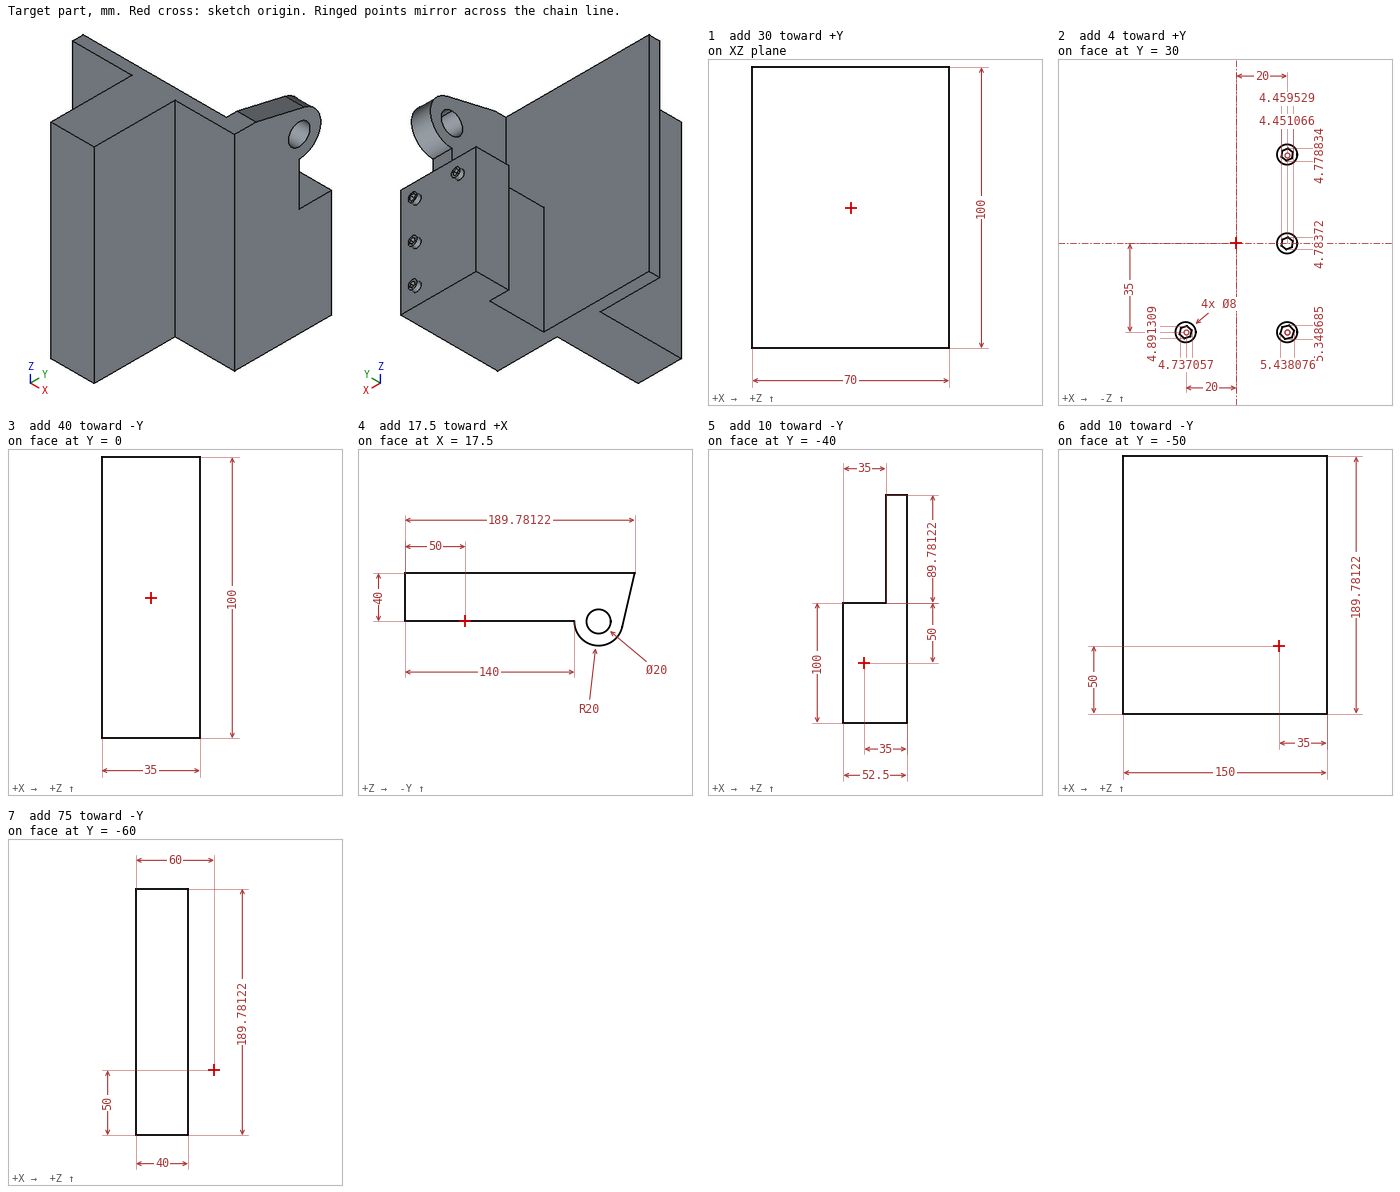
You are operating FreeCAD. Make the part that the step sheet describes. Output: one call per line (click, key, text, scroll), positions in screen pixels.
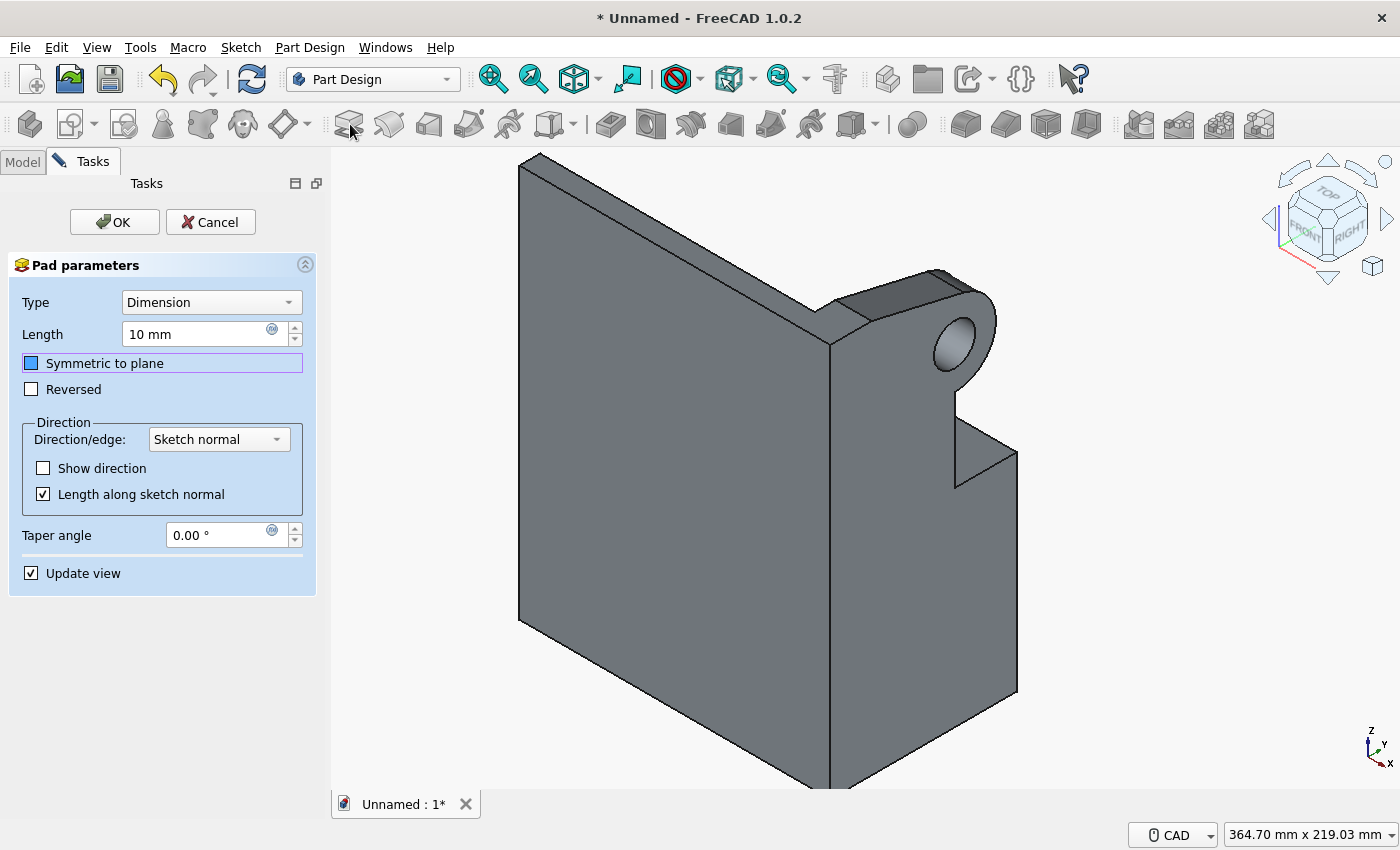
click(115, 222)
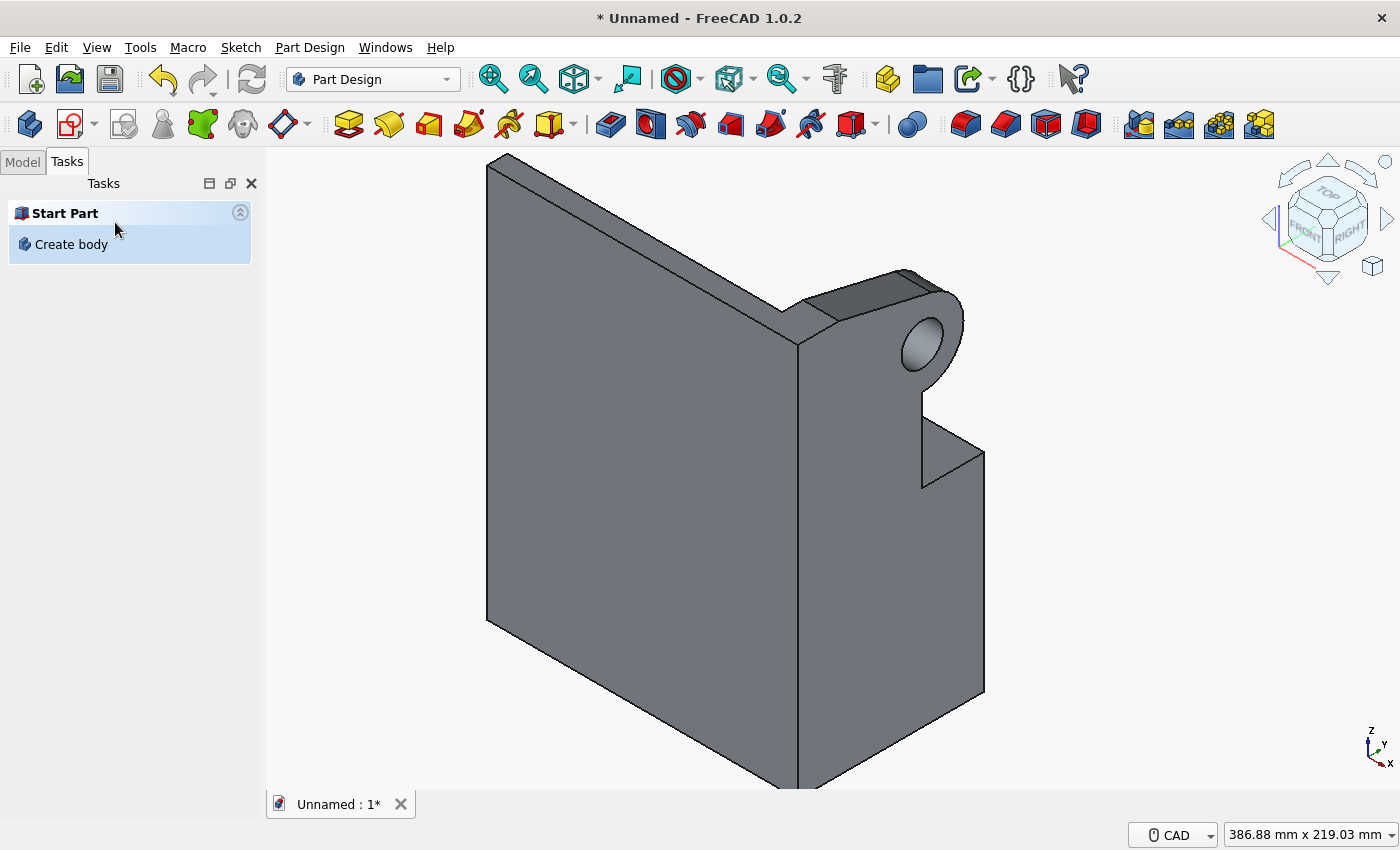
click(494, 80)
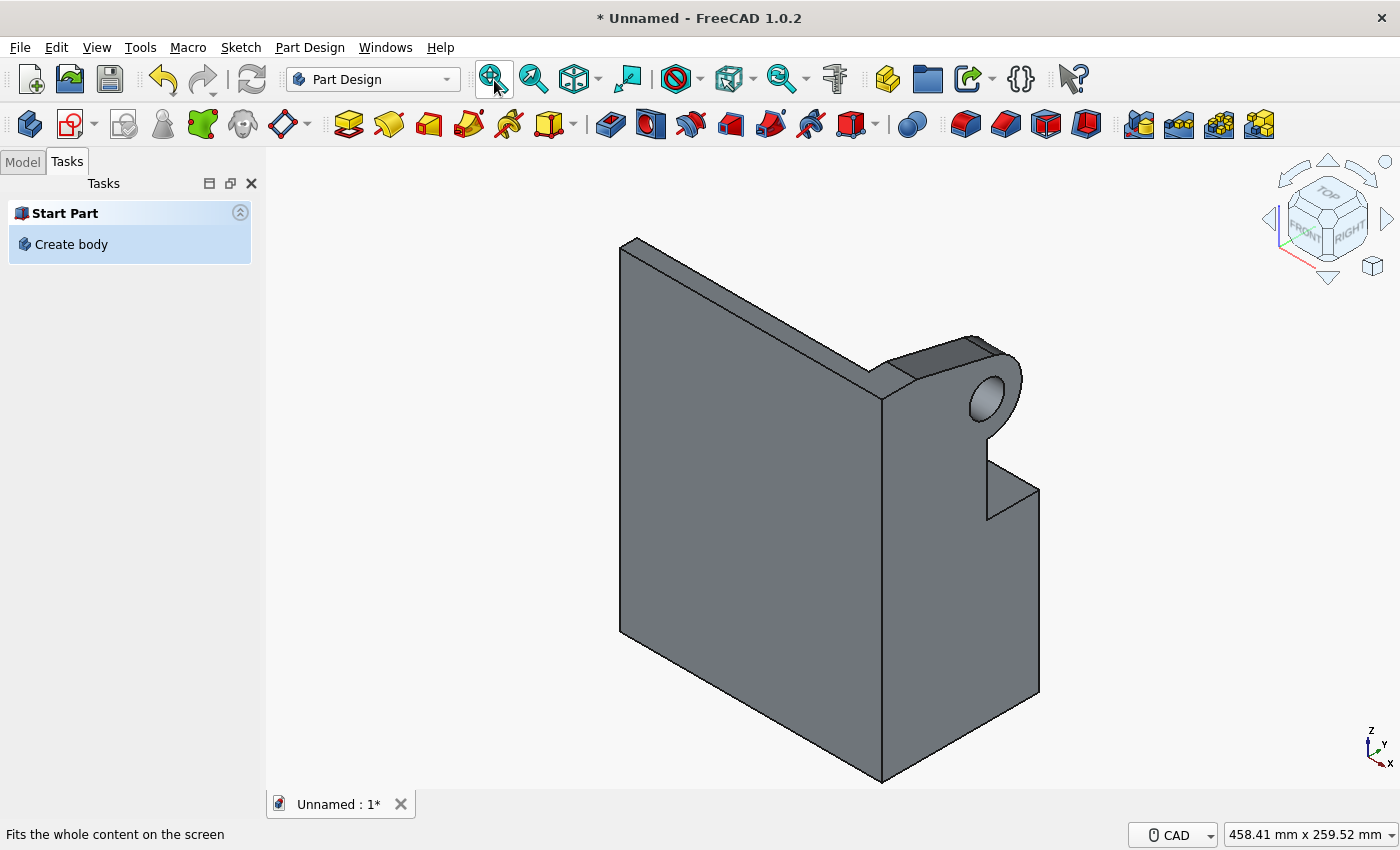
click(751, 514)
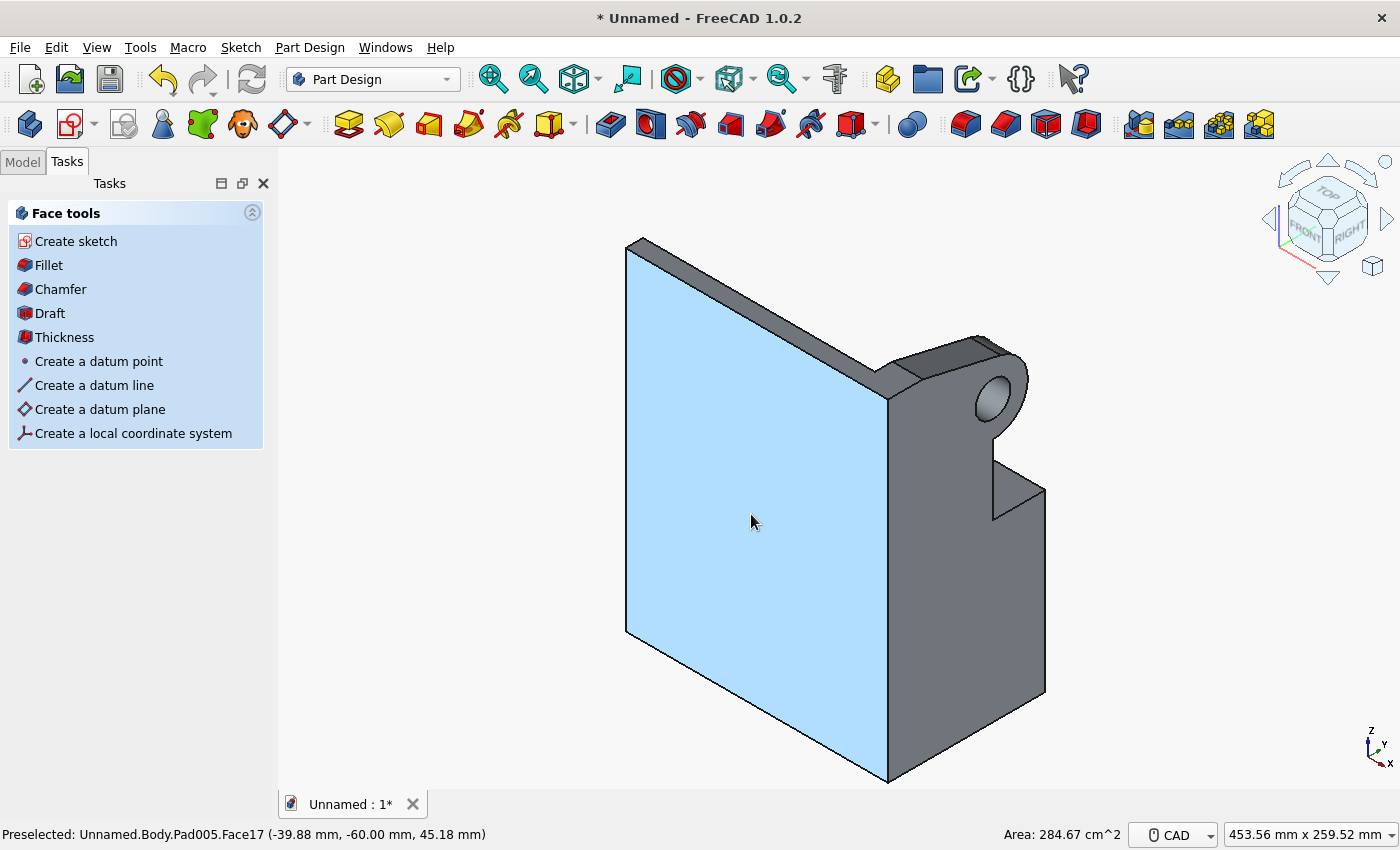
click(70, 124)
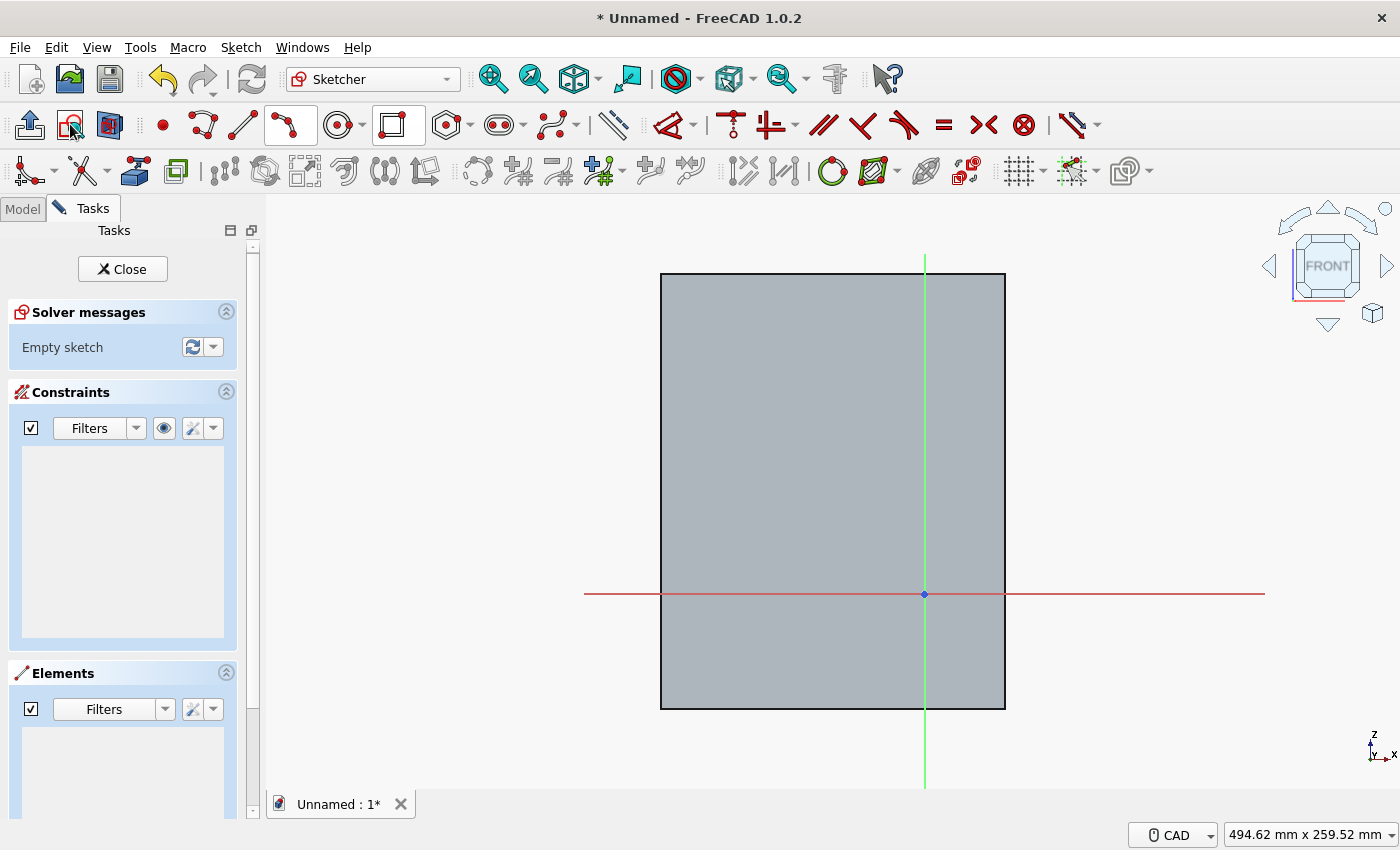
click(392, 126)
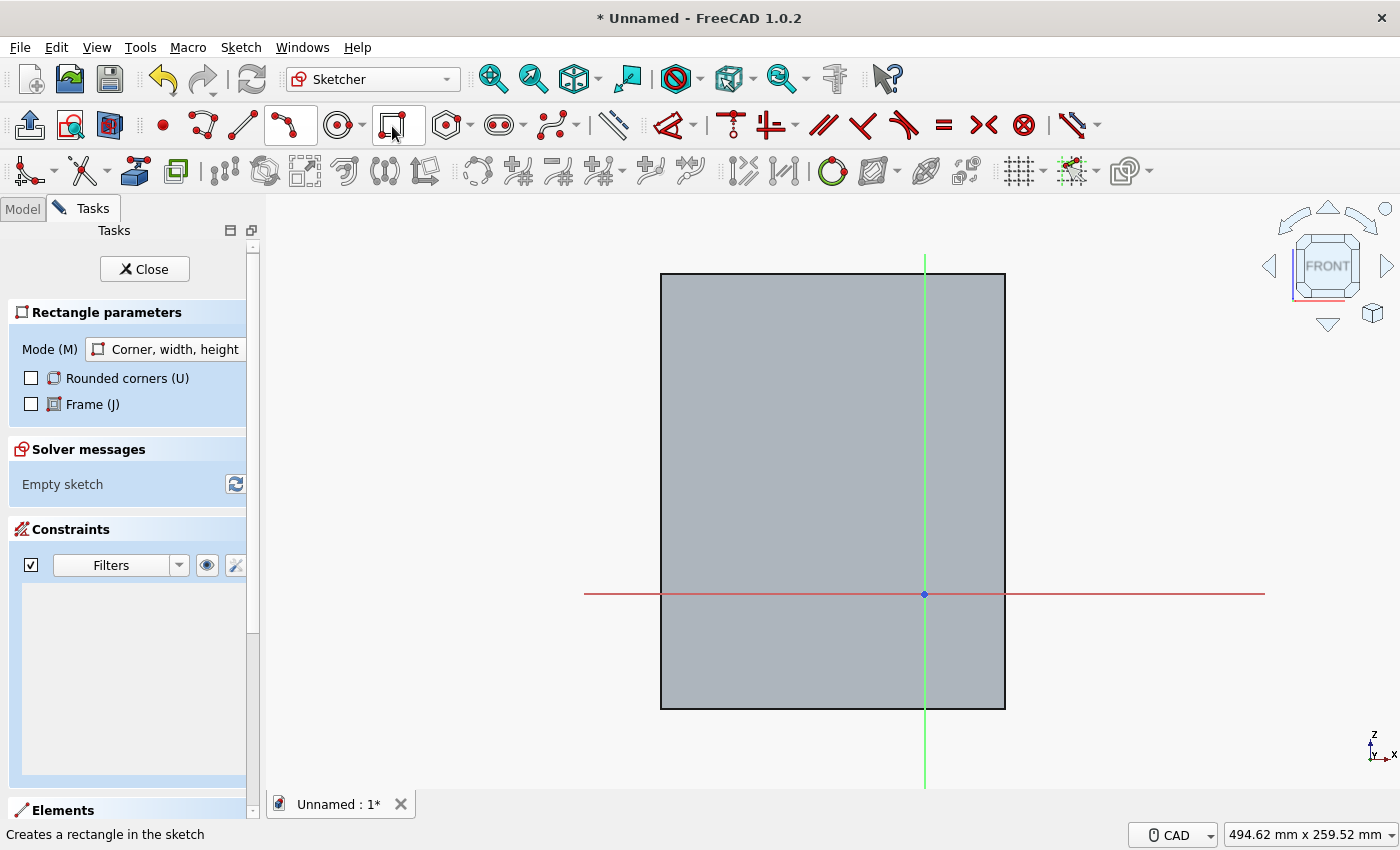
click(787, 274)
move(879, 709)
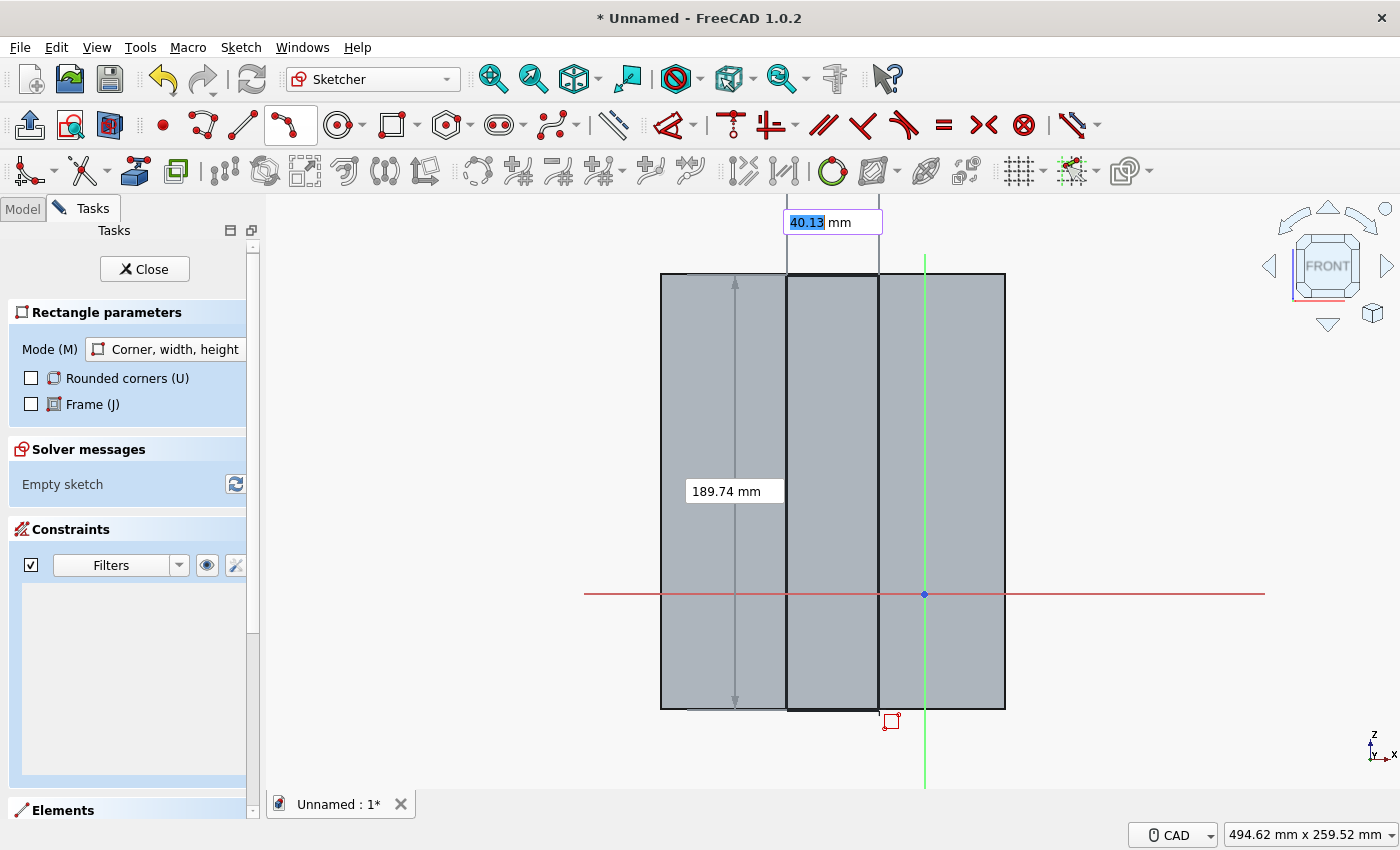
text(40)
key(Tab)
text(189.78122)
key(Return)
key(Escape)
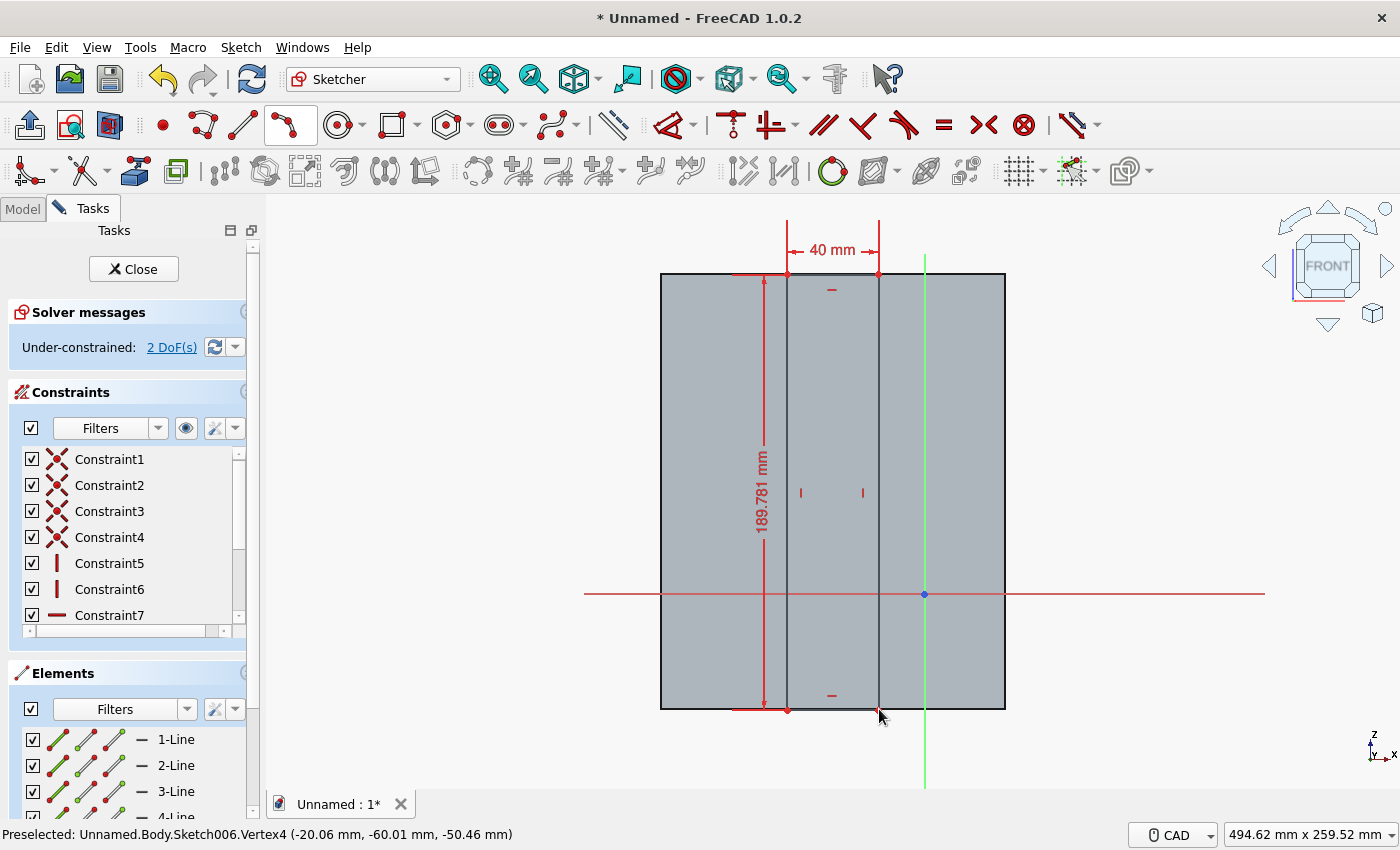
click(668, 126)